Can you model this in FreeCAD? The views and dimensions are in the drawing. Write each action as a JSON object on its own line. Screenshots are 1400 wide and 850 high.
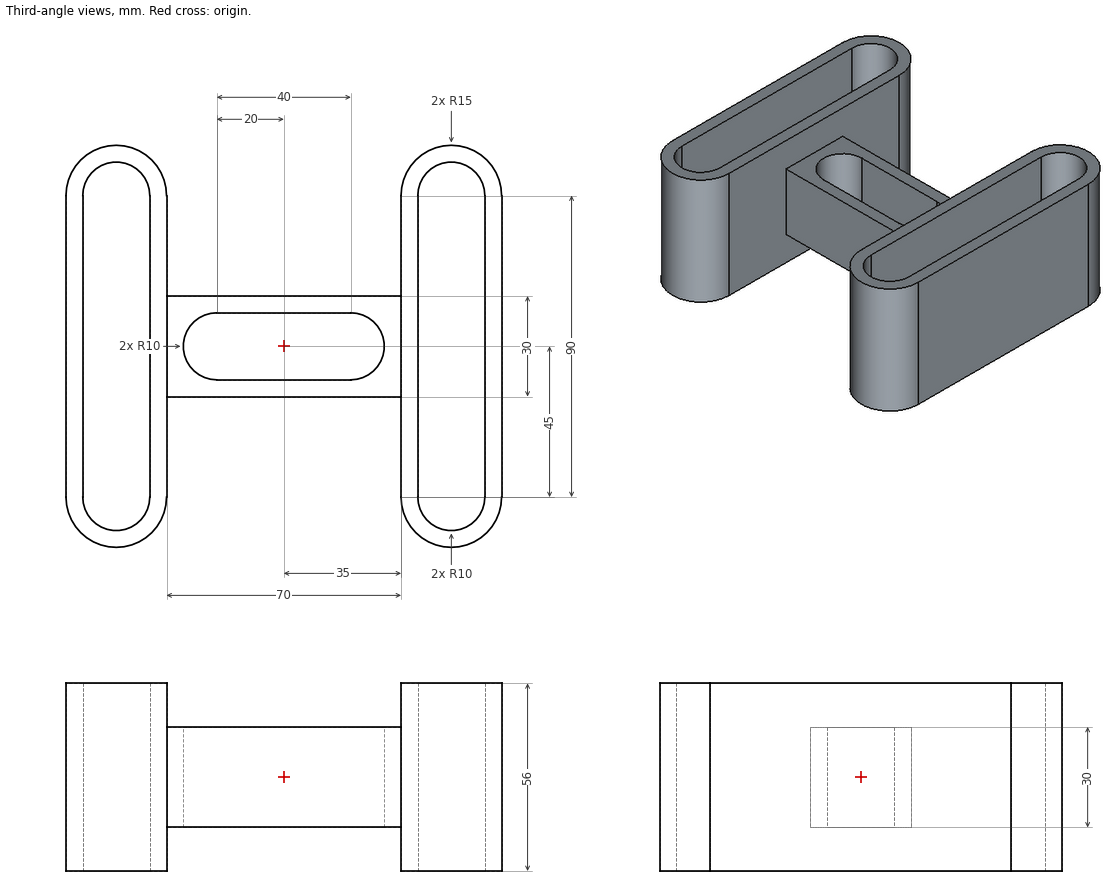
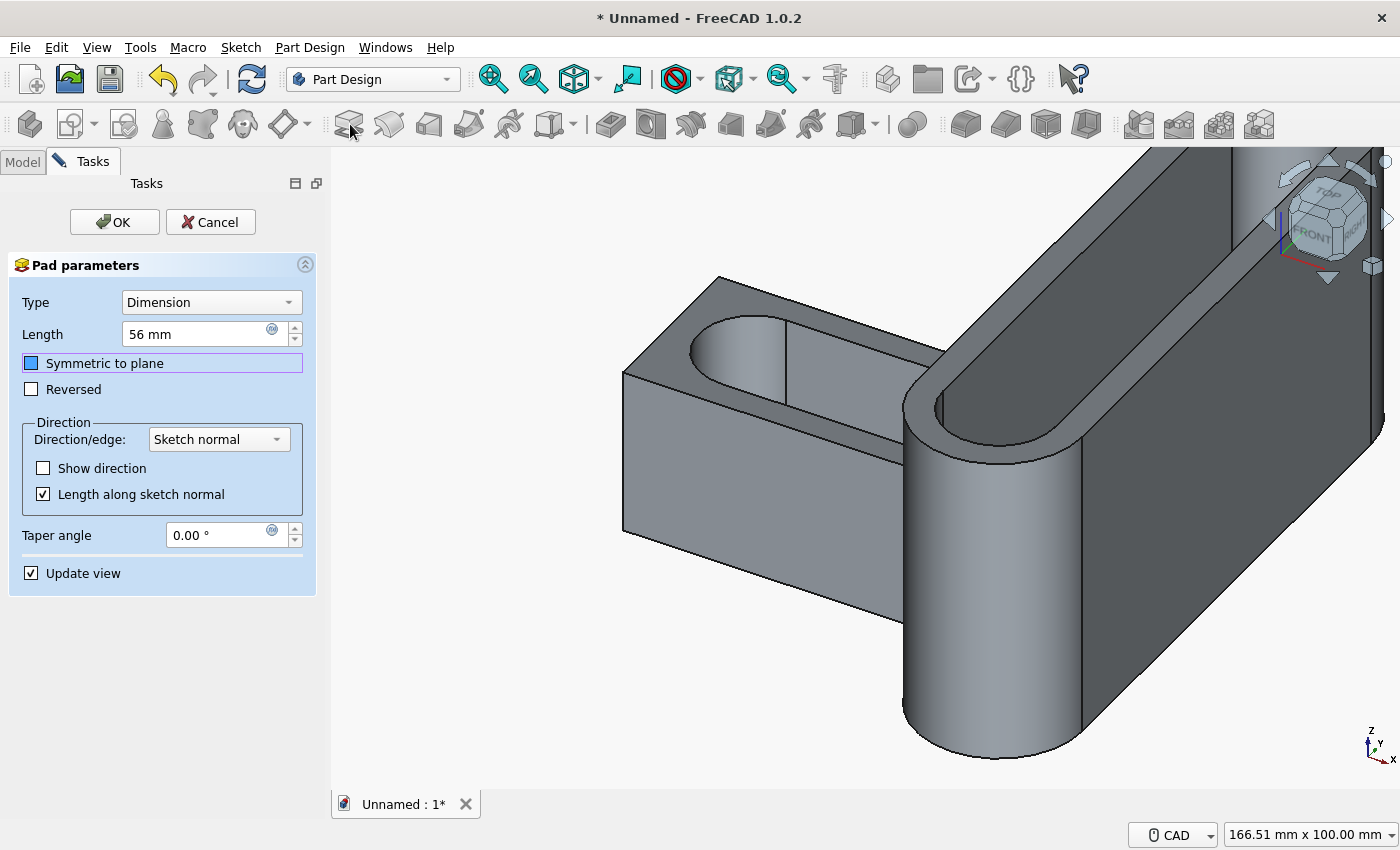
{"action": "left_click", "coordinate": [30, 363]}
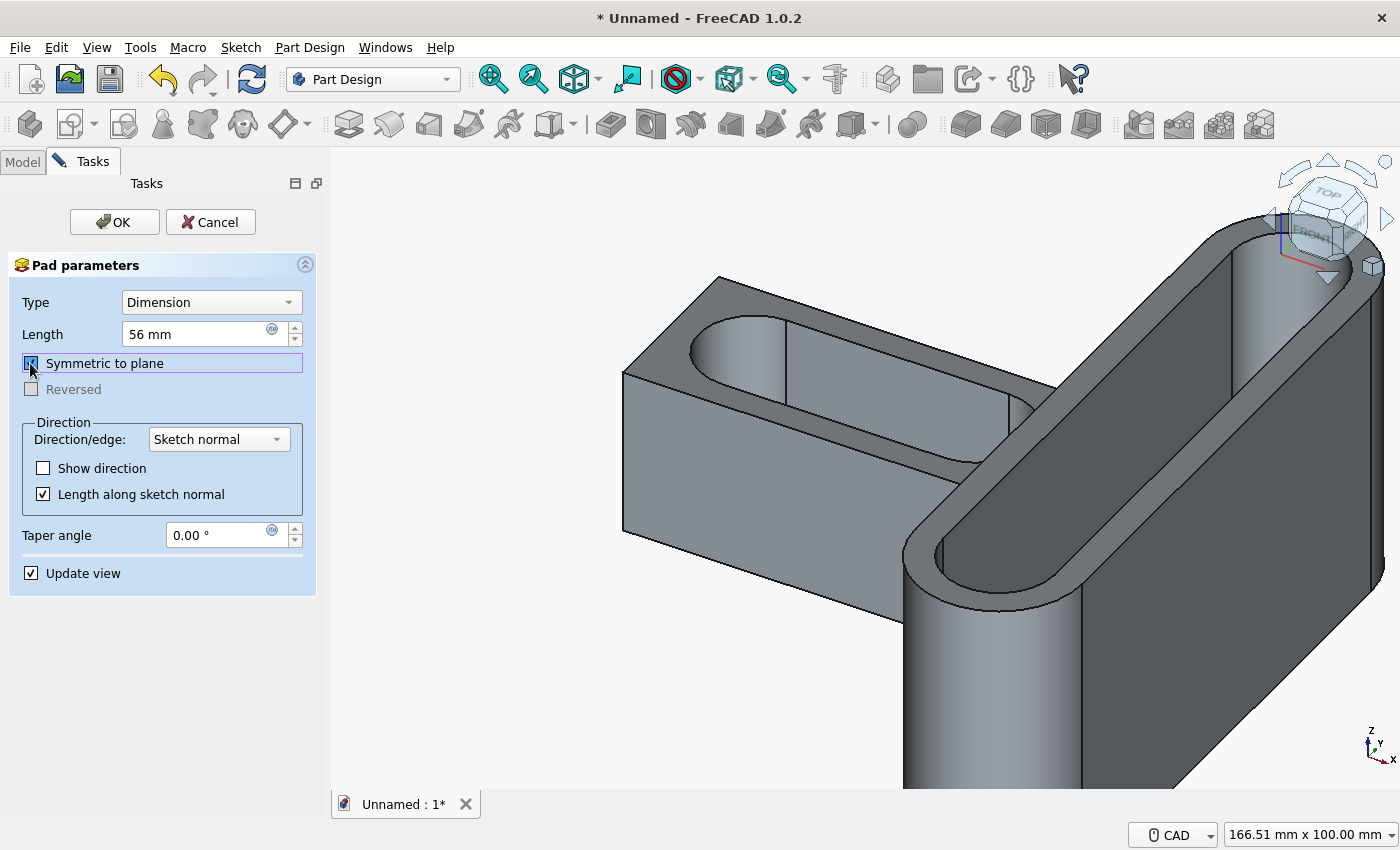
{"action": "left_click", "coordinate": [115, 222]}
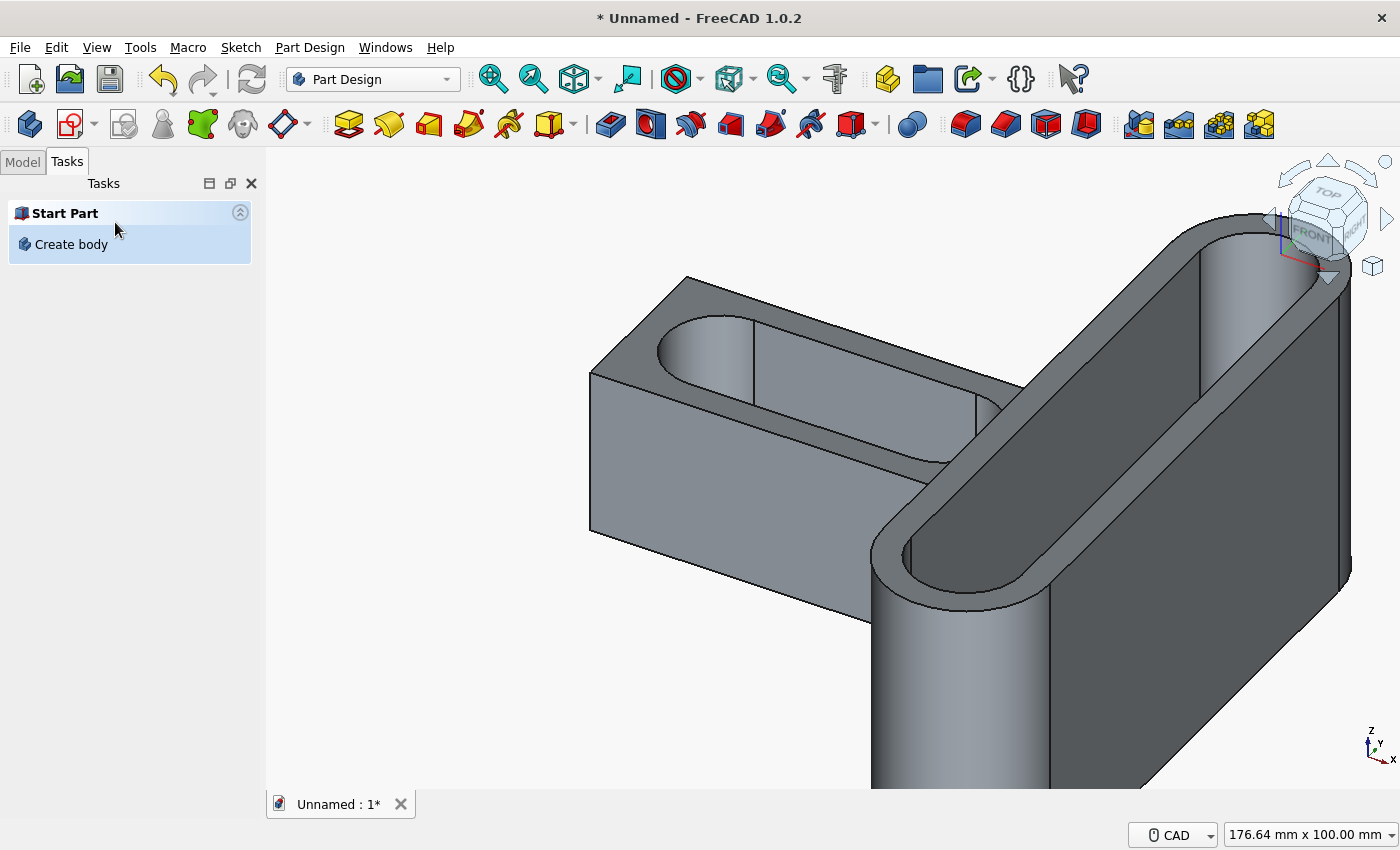
{"action": "key", "text": "v f"}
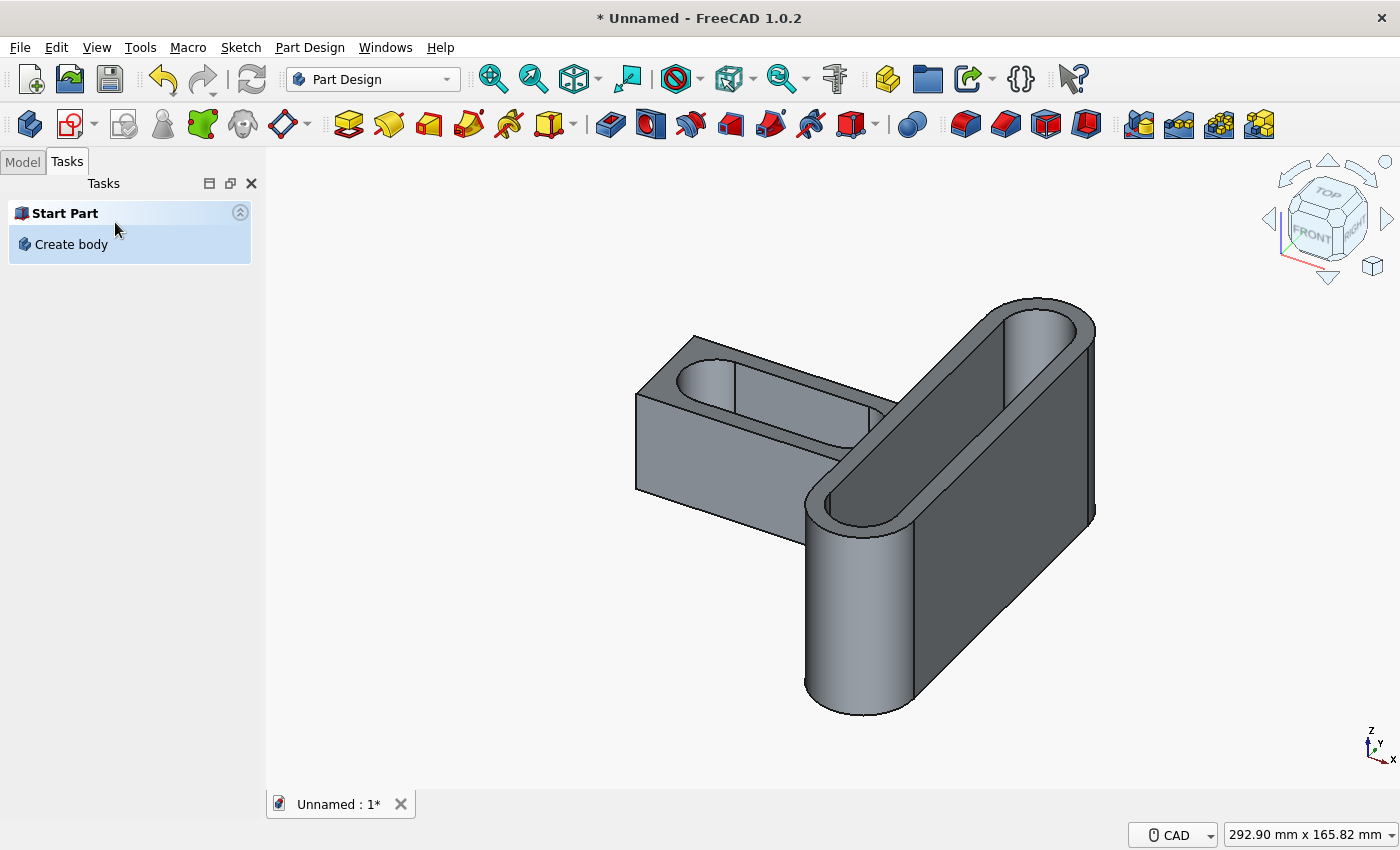
{"action": "left_click", "coordinate": [23, 161]}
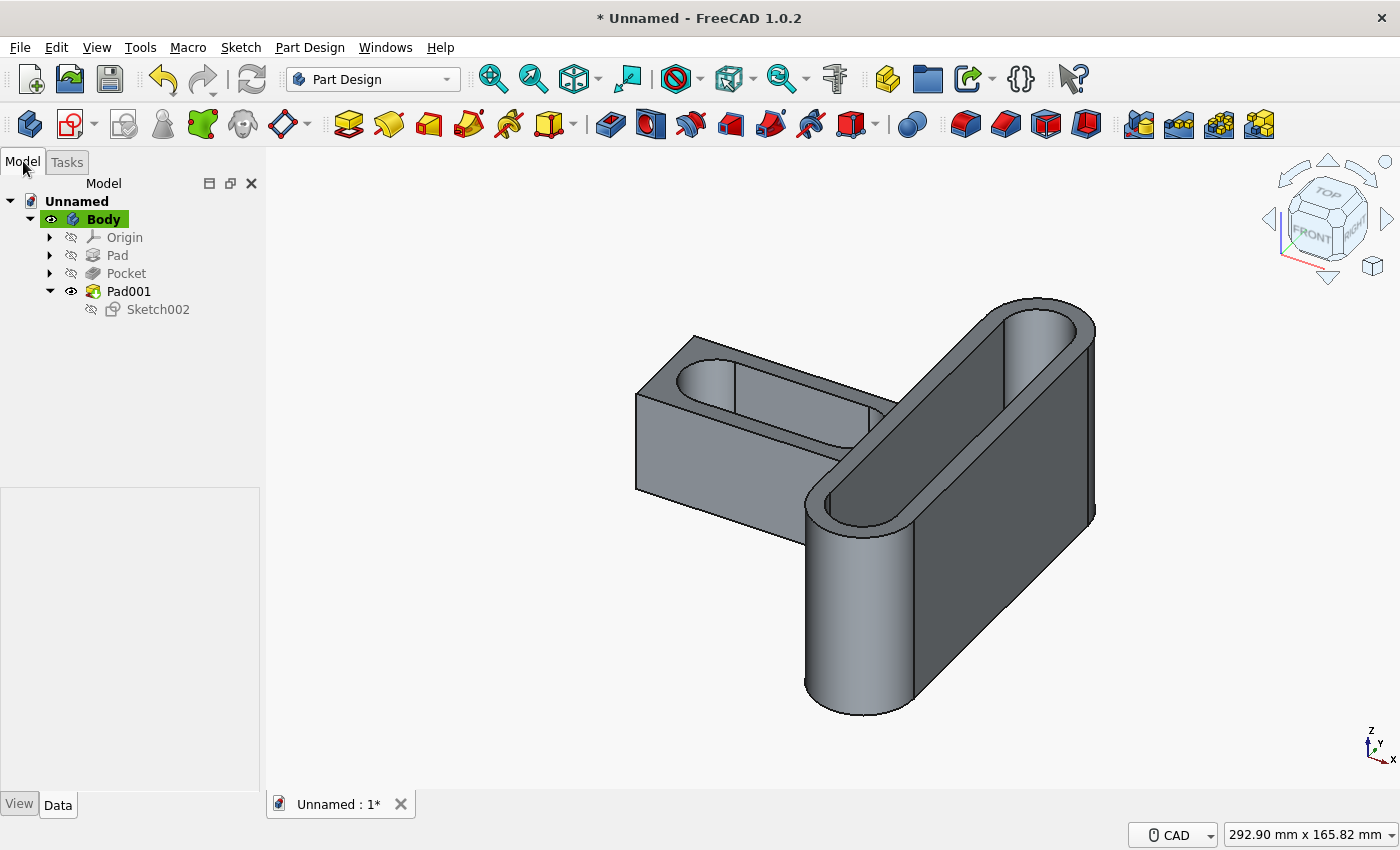
{"action": "left_click", "coordinate": [116, 291]}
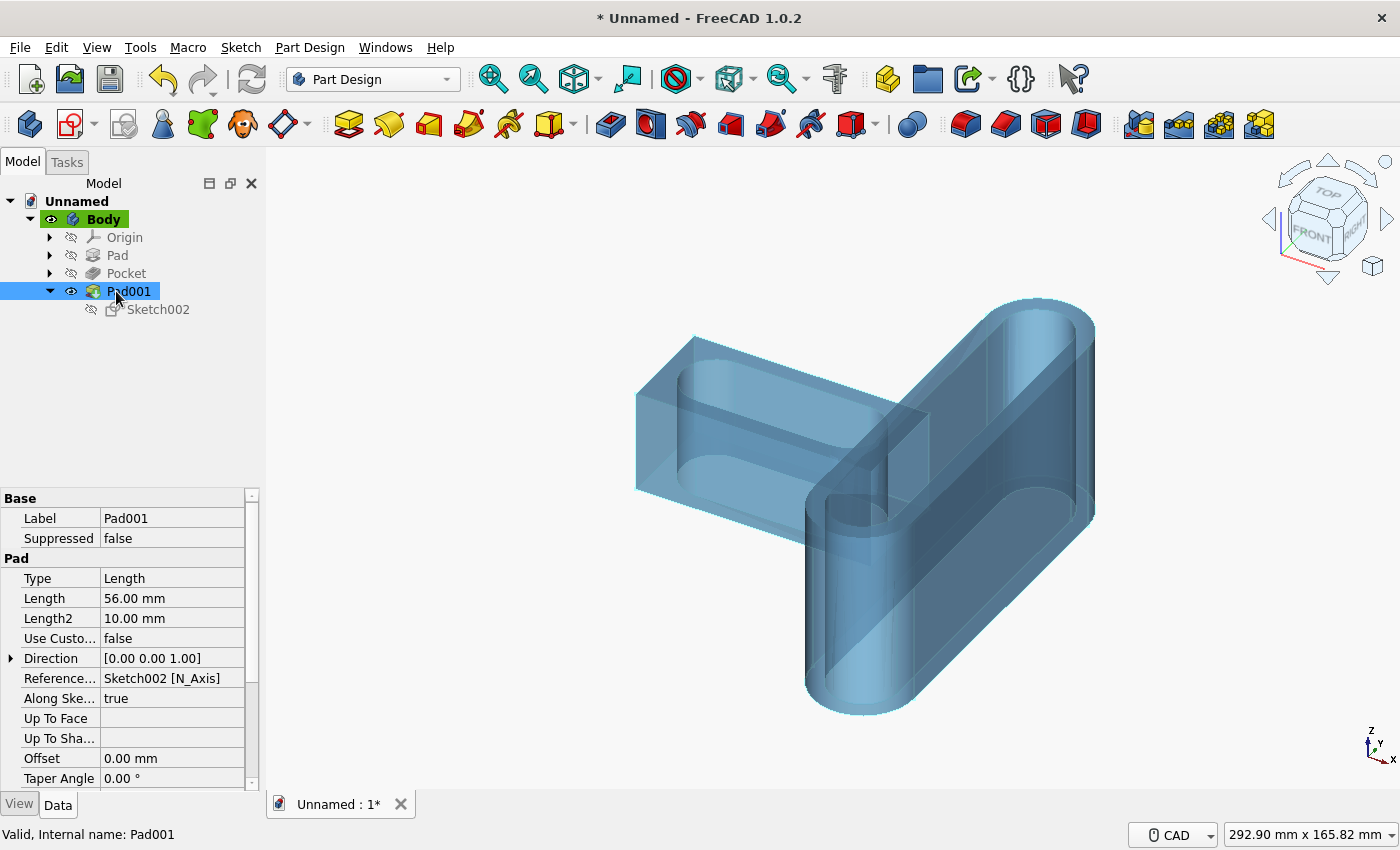
{"action": "left_click", "coordinate": [1140, 124]}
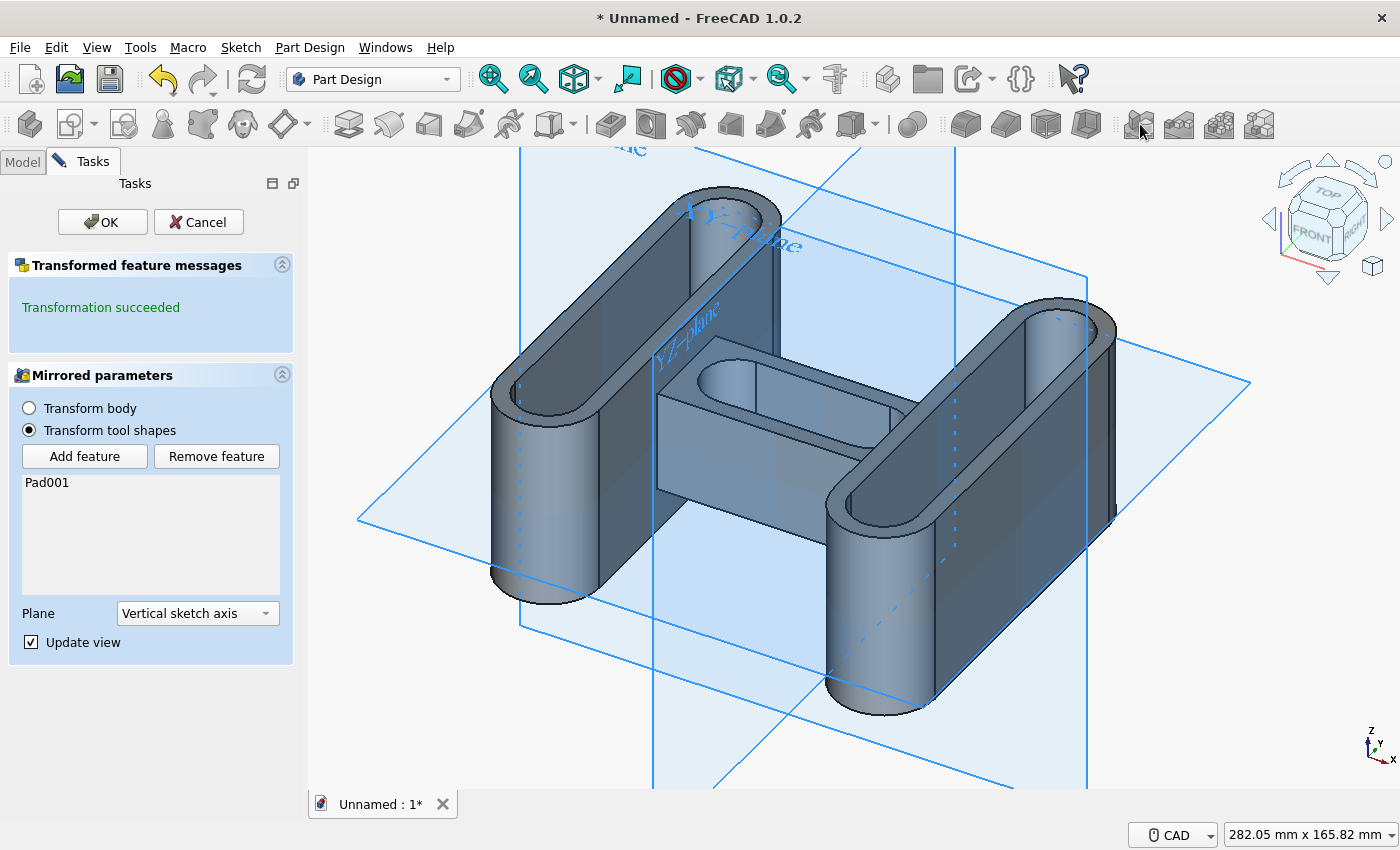
{"action": "left_click", "coordinate": [198, 614]}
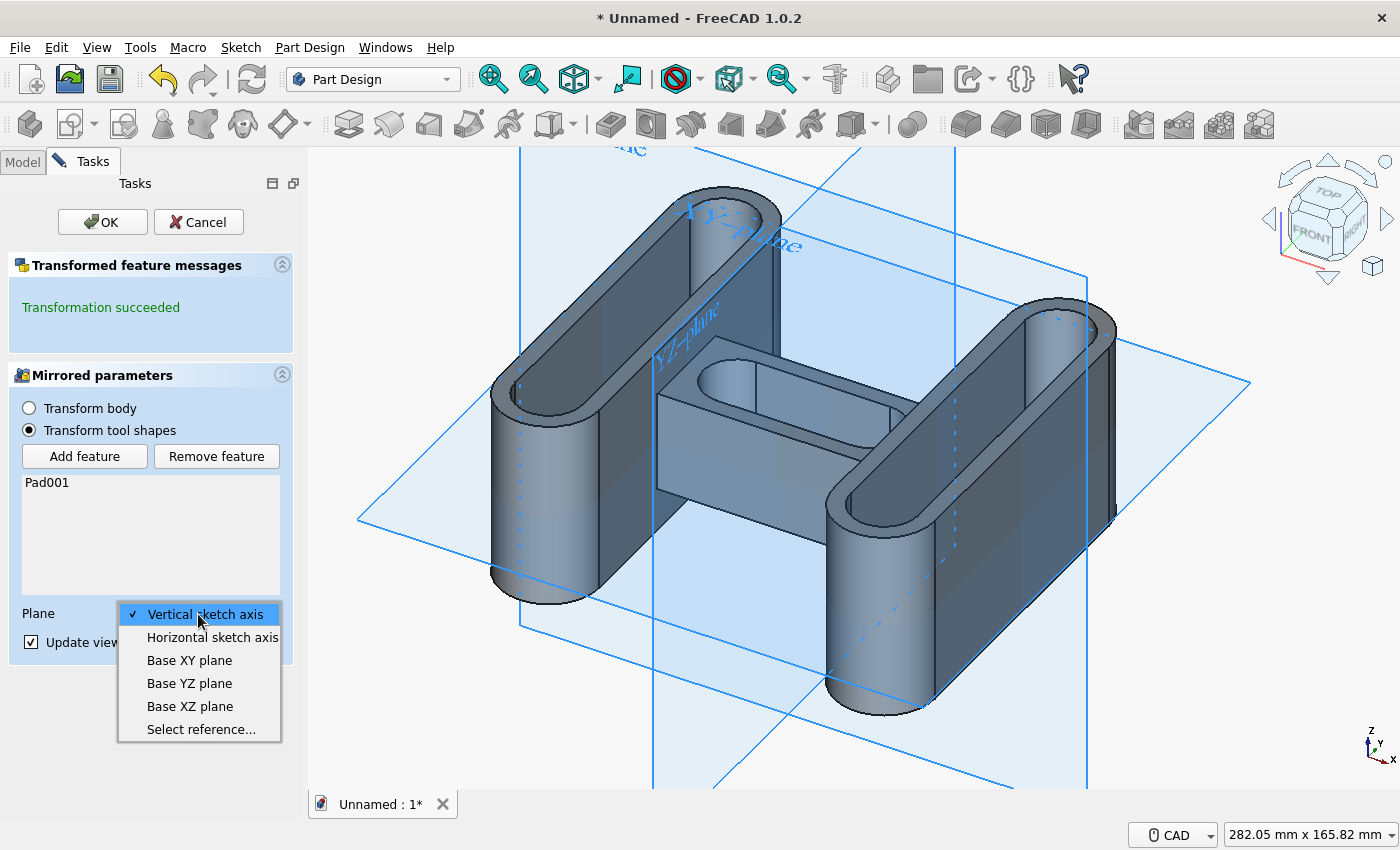
{"action": "left_click", "coordinate": [198, 684]}